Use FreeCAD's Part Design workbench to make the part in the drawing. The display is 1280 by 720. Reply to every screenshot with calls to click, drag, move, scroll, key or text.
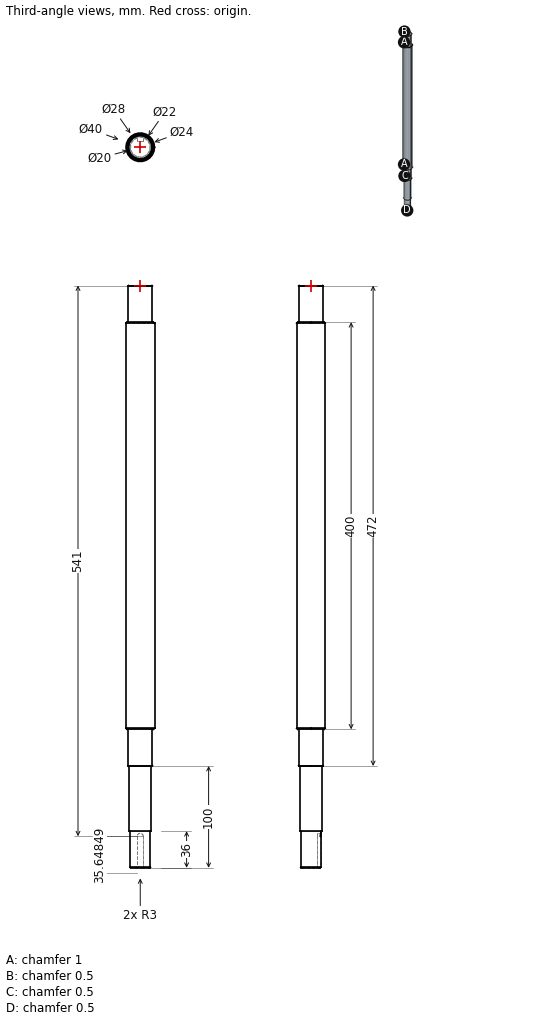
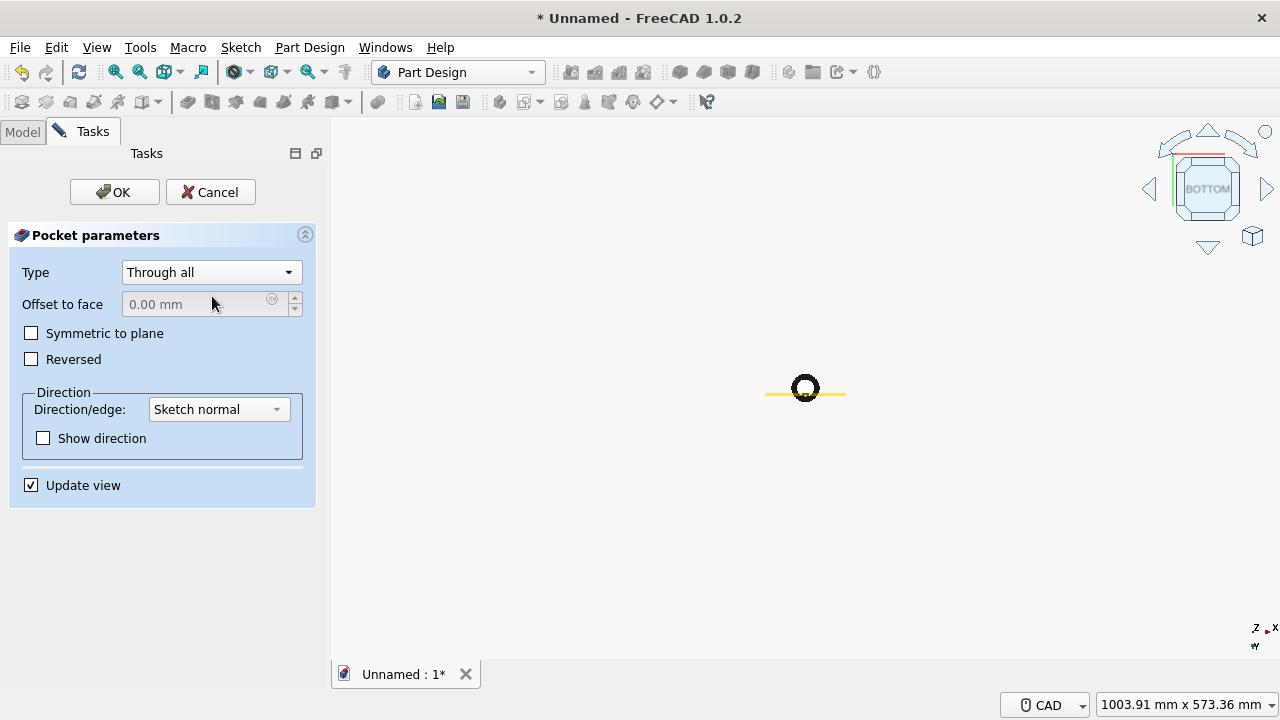
click(115, 192)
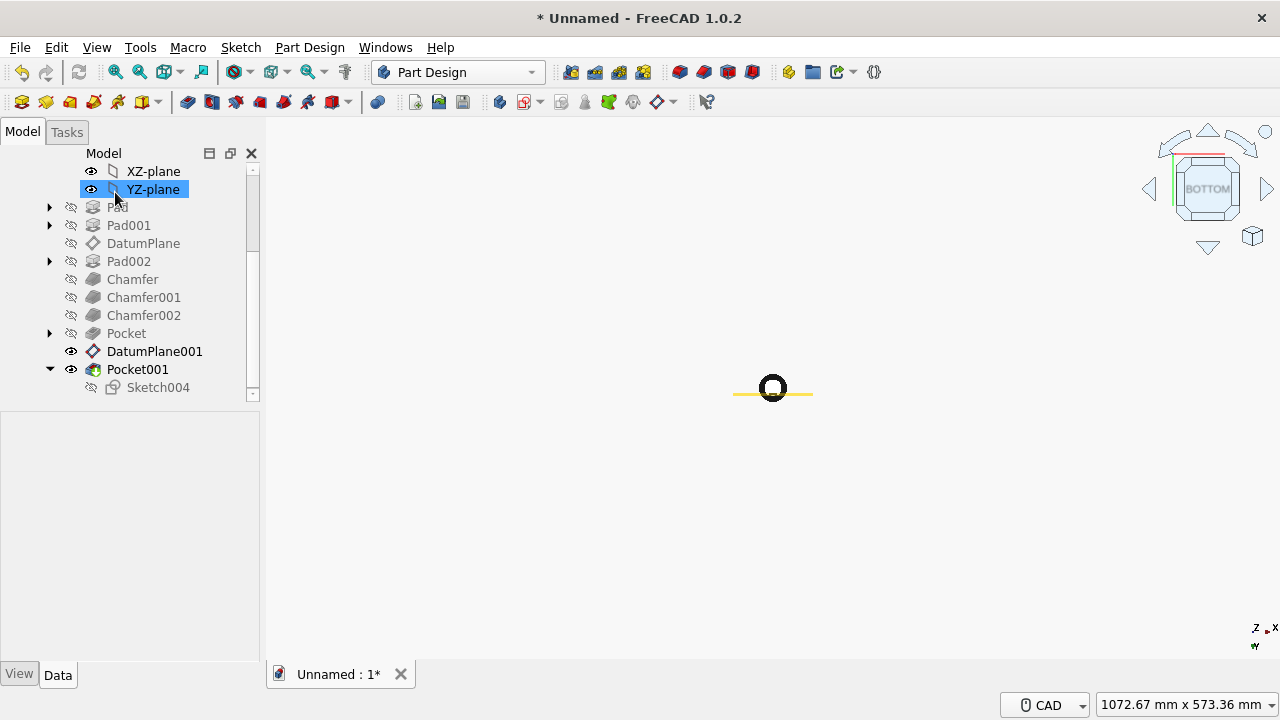
click(116, 351)
key(space)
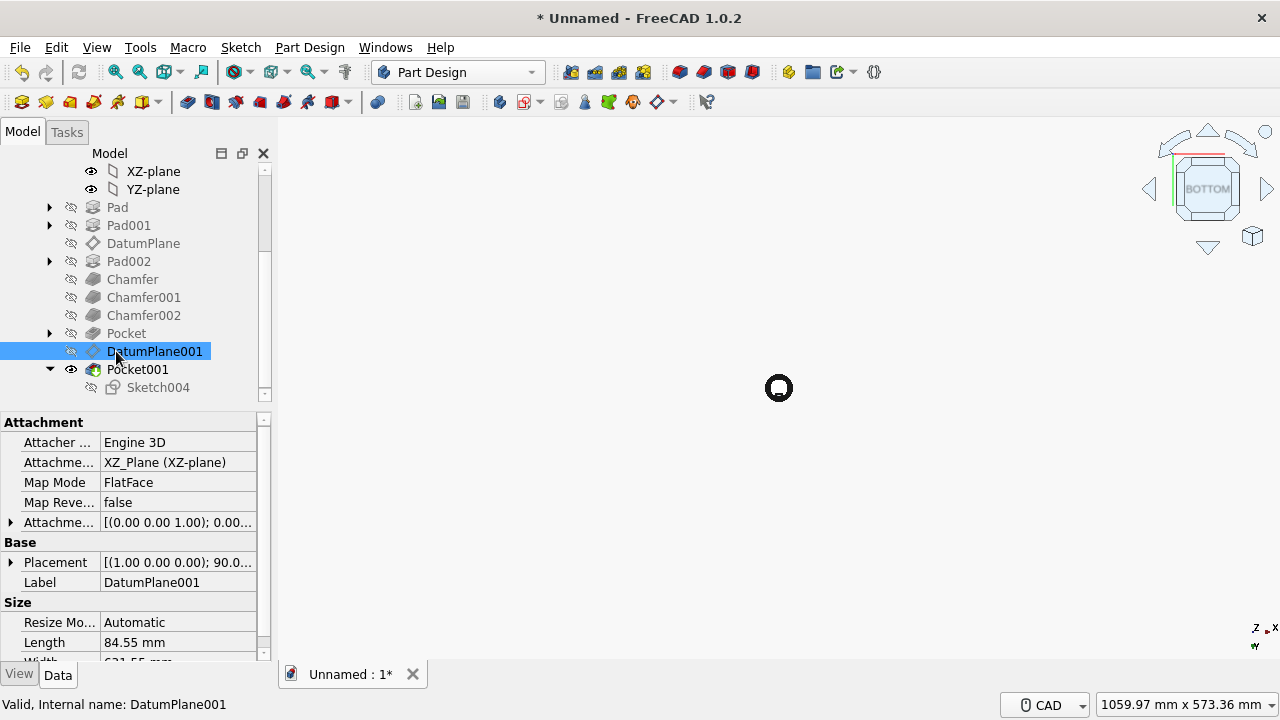
key(v)
key(f)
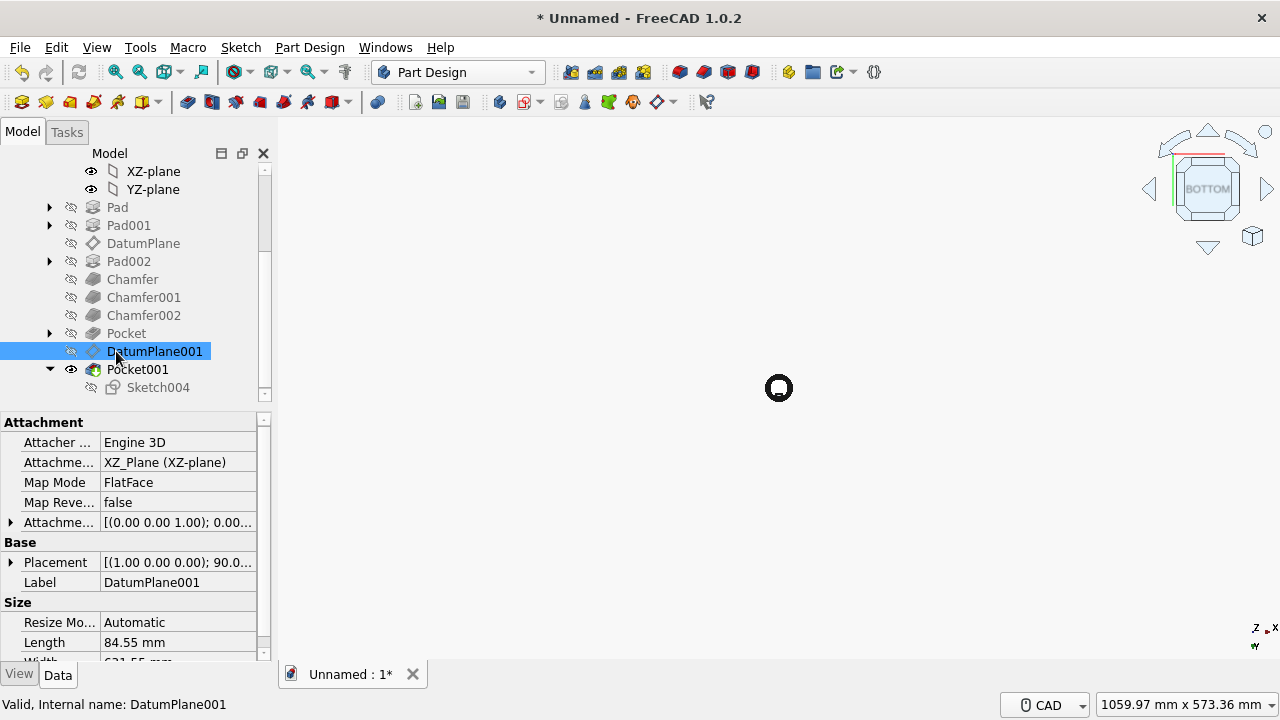
click(773, 379)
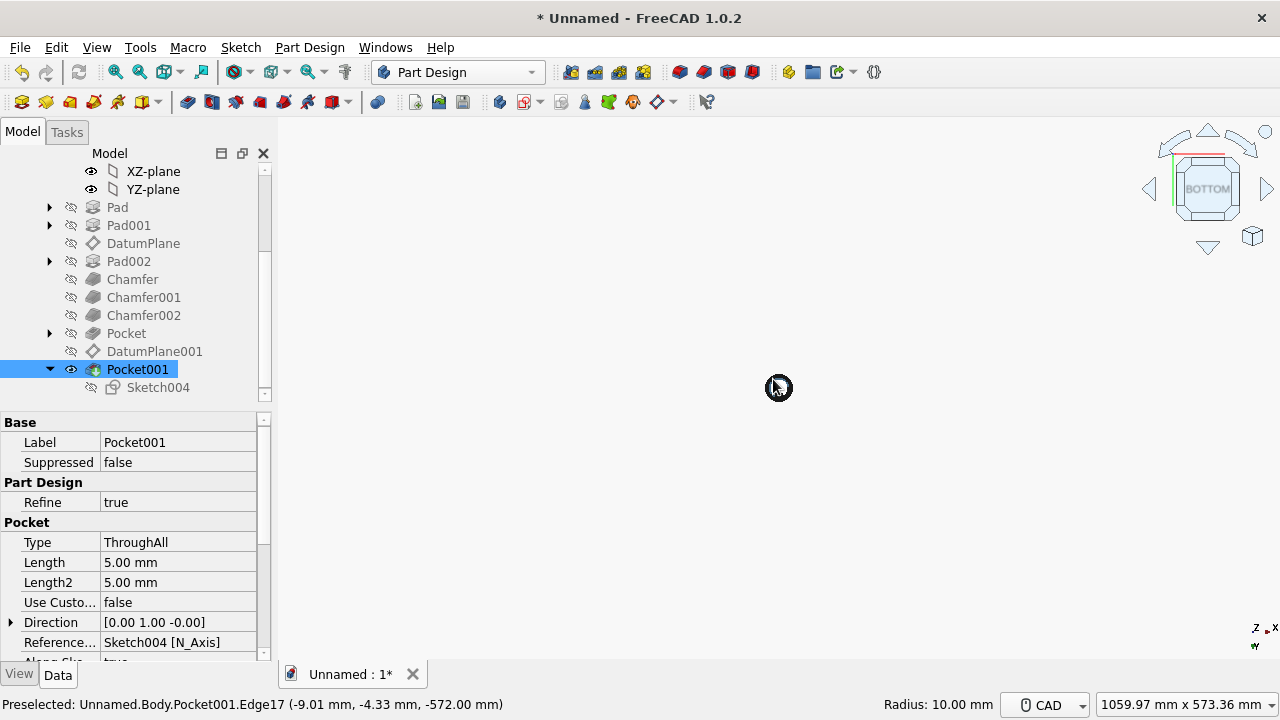
click(704, 72)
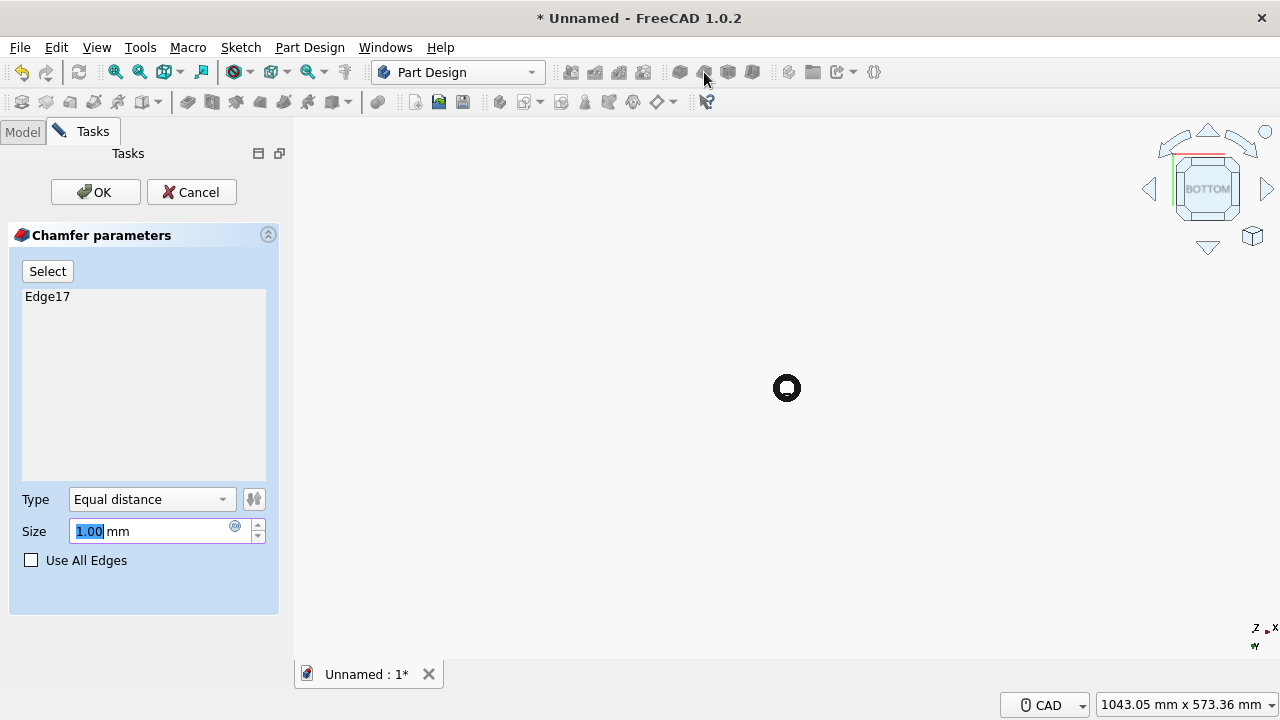
text(0.5)
key(Tab)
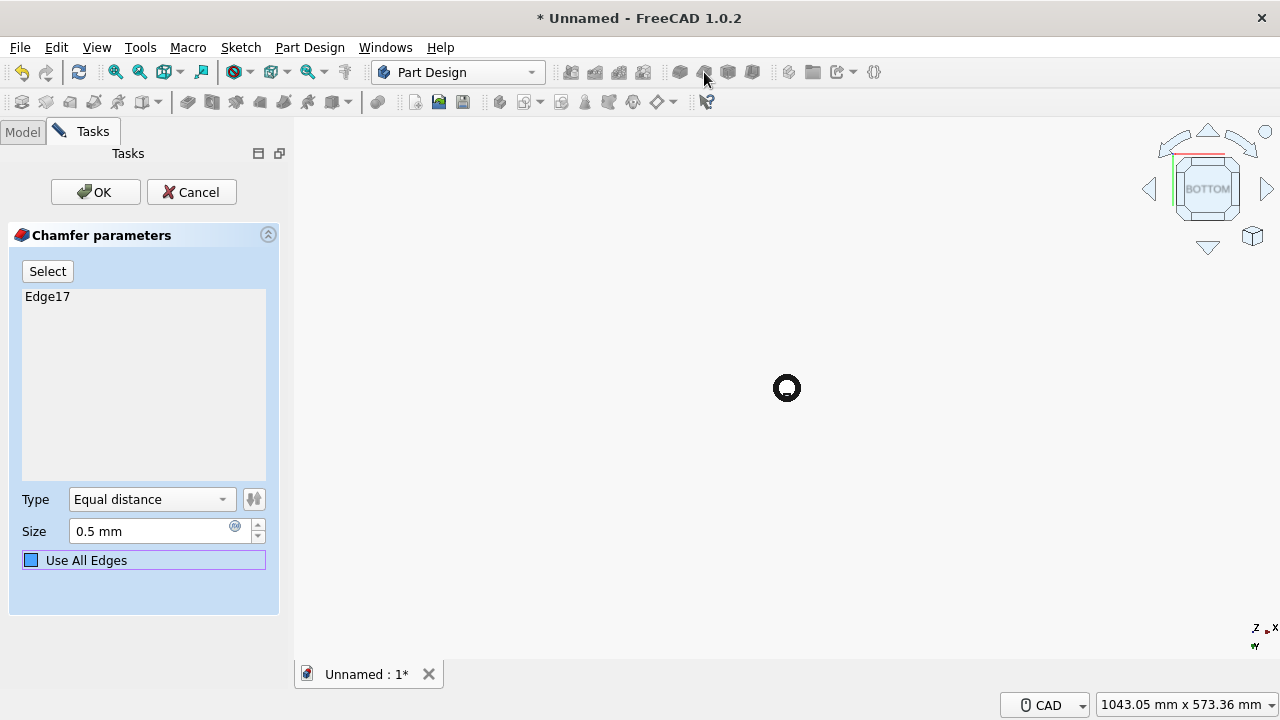
click(96, 192)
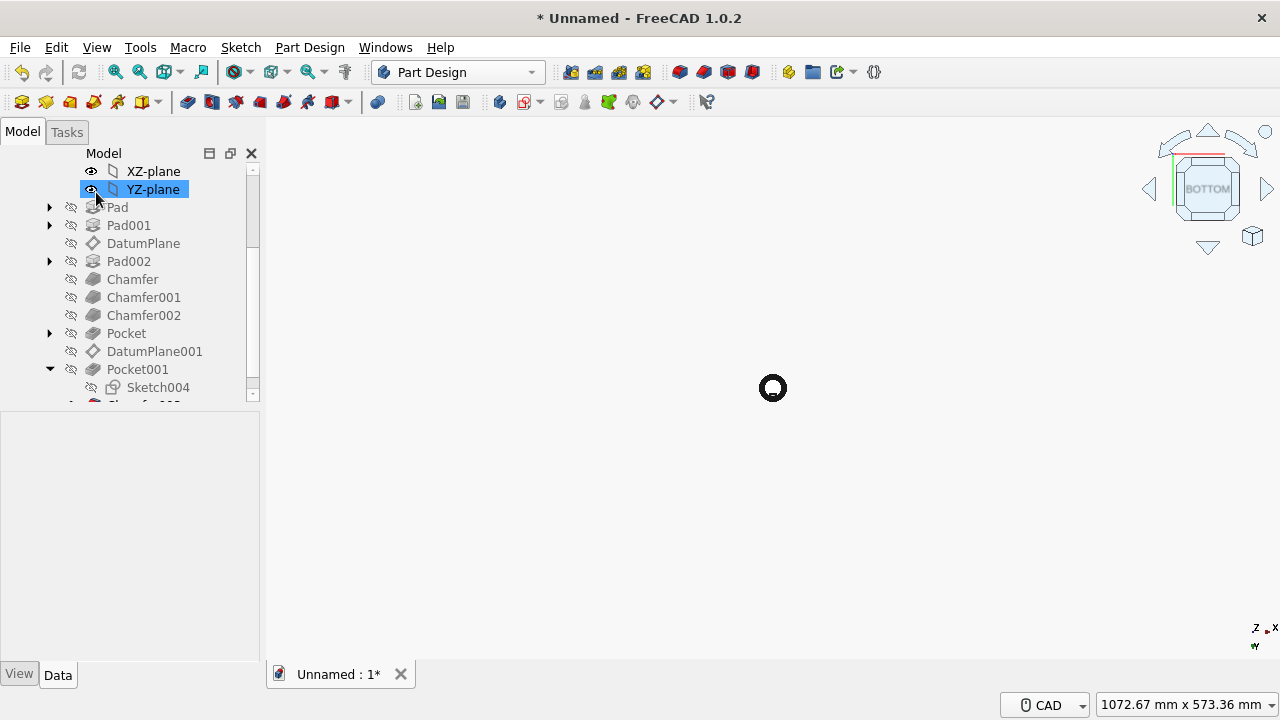
key(0)